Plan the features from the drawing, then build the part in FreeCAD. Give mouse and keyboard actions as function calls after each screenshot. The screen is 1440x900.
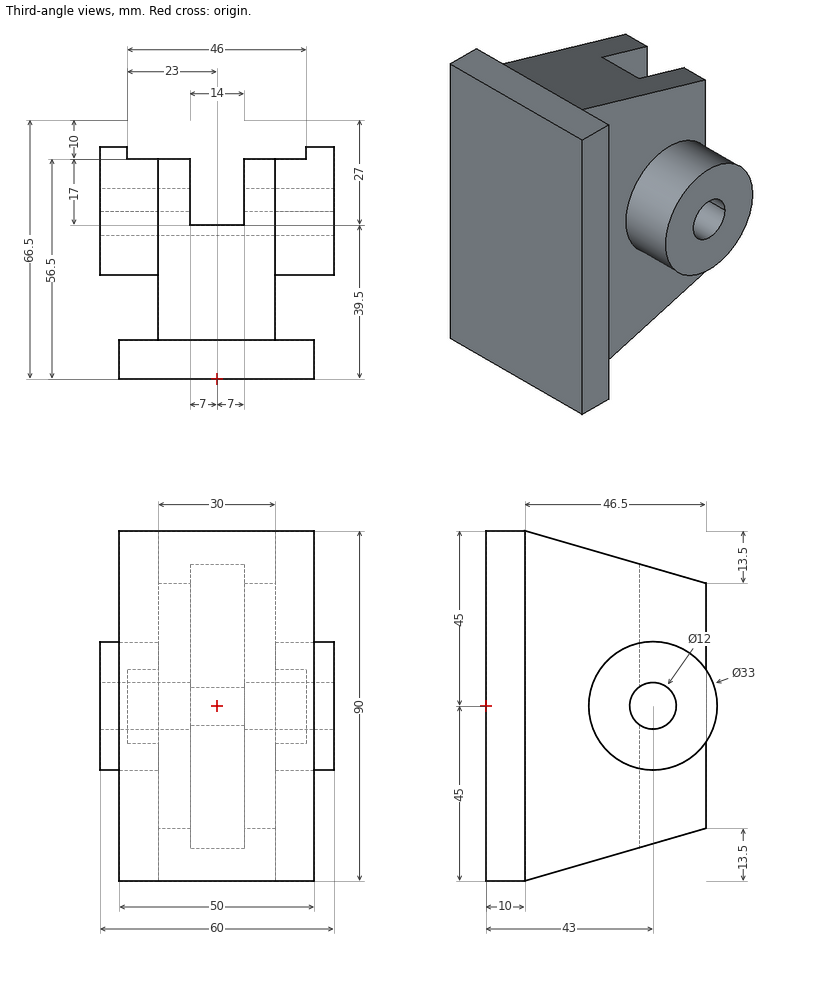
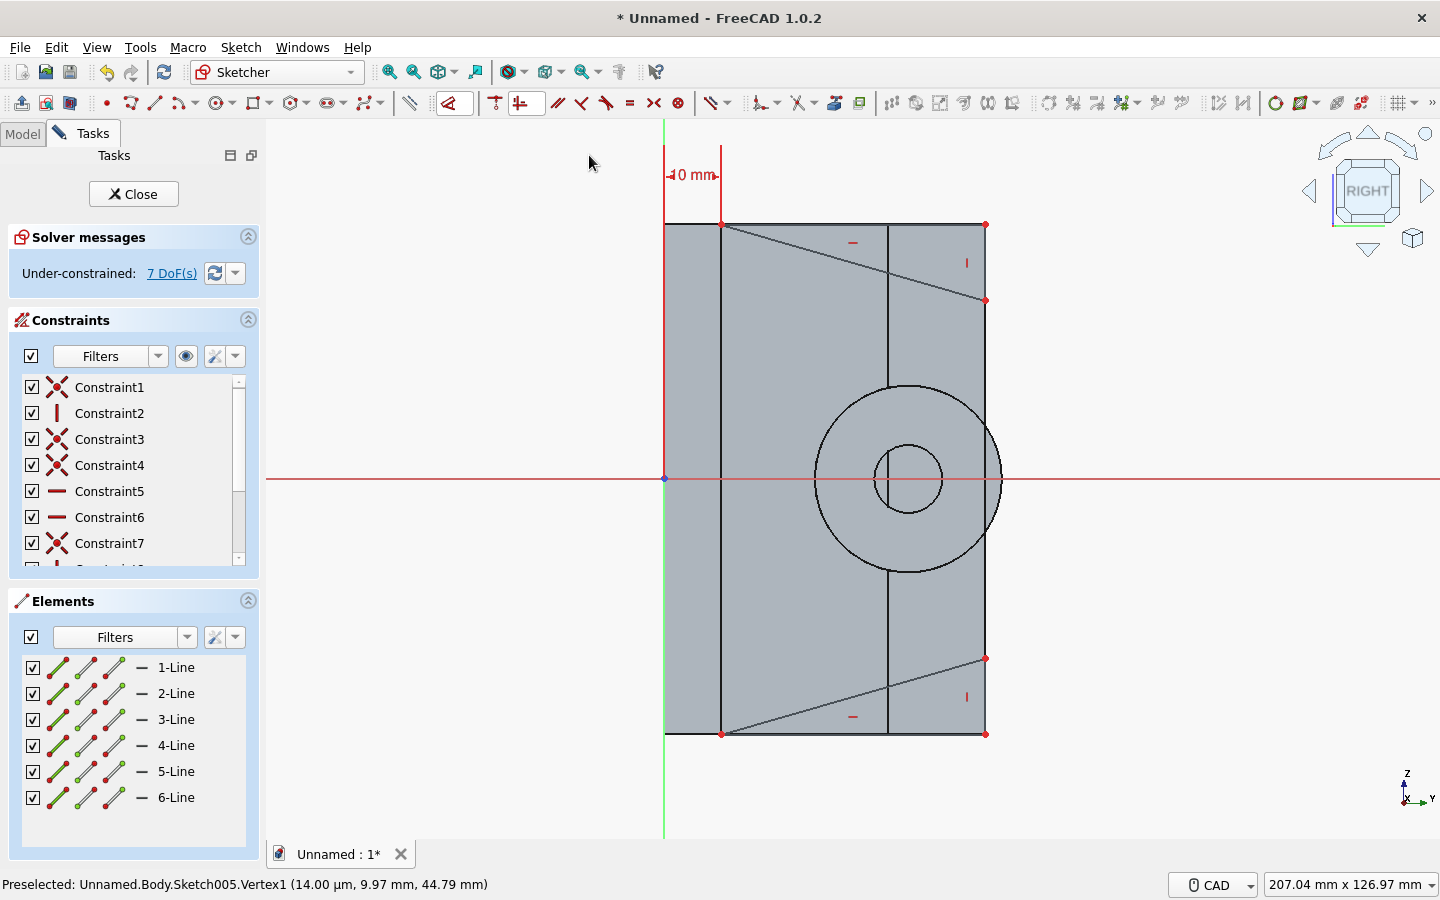
click(721, 225)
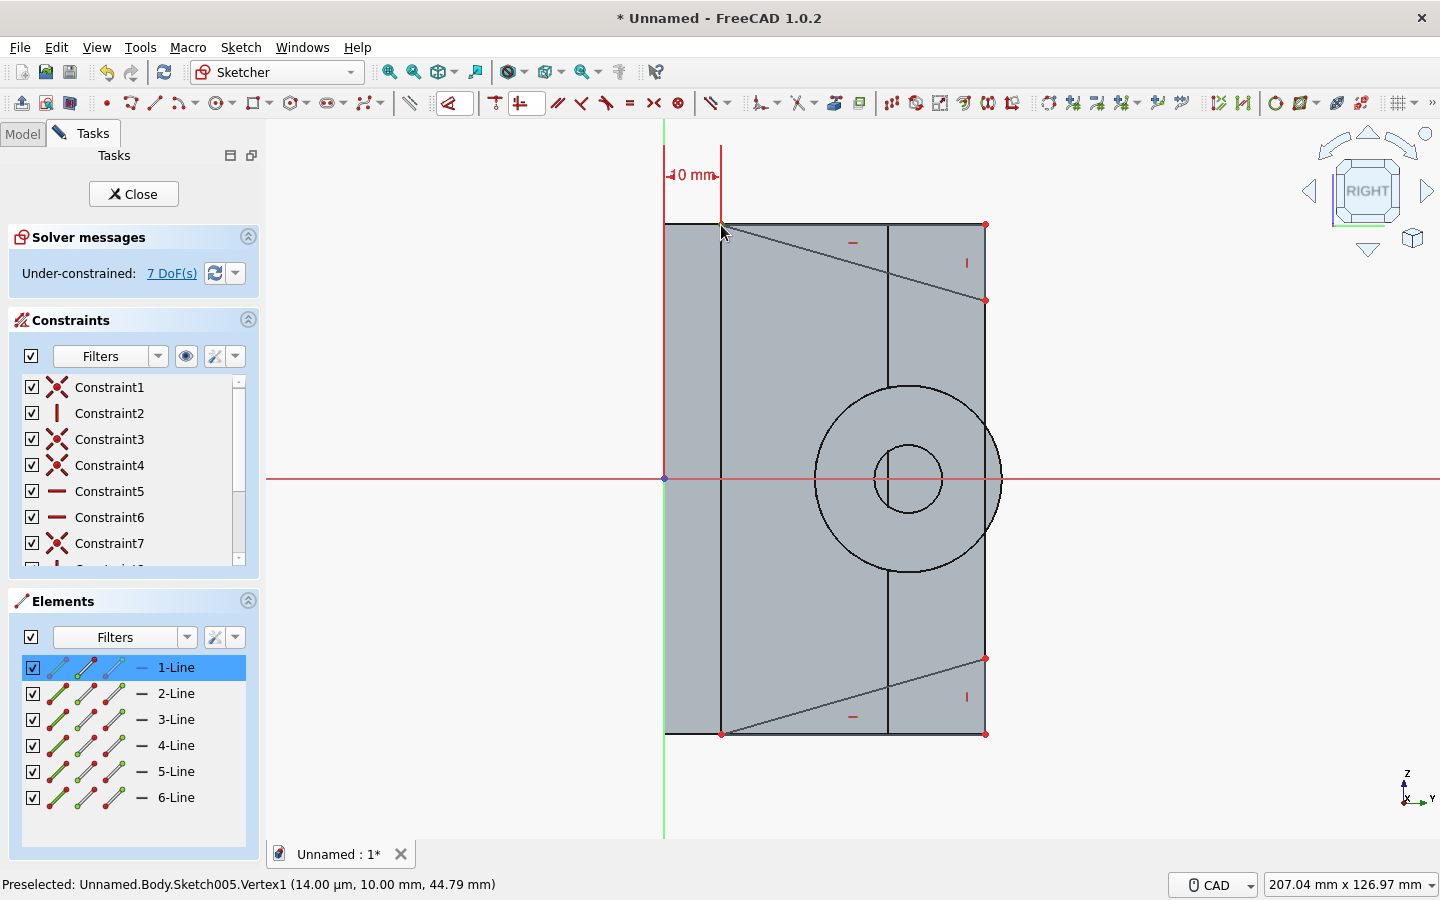
click(468, 104)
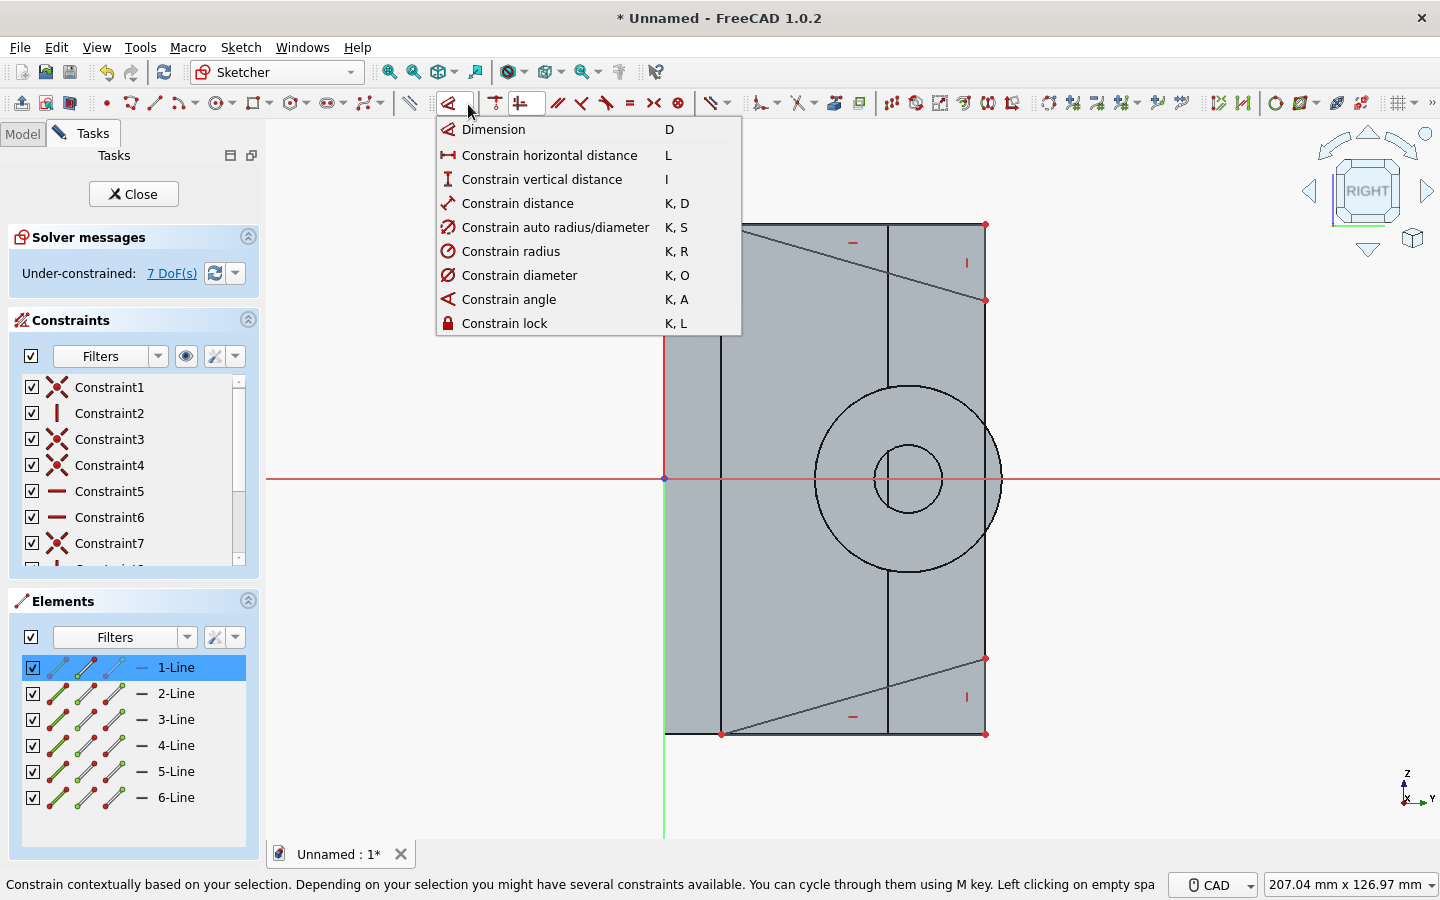
click(589, 179)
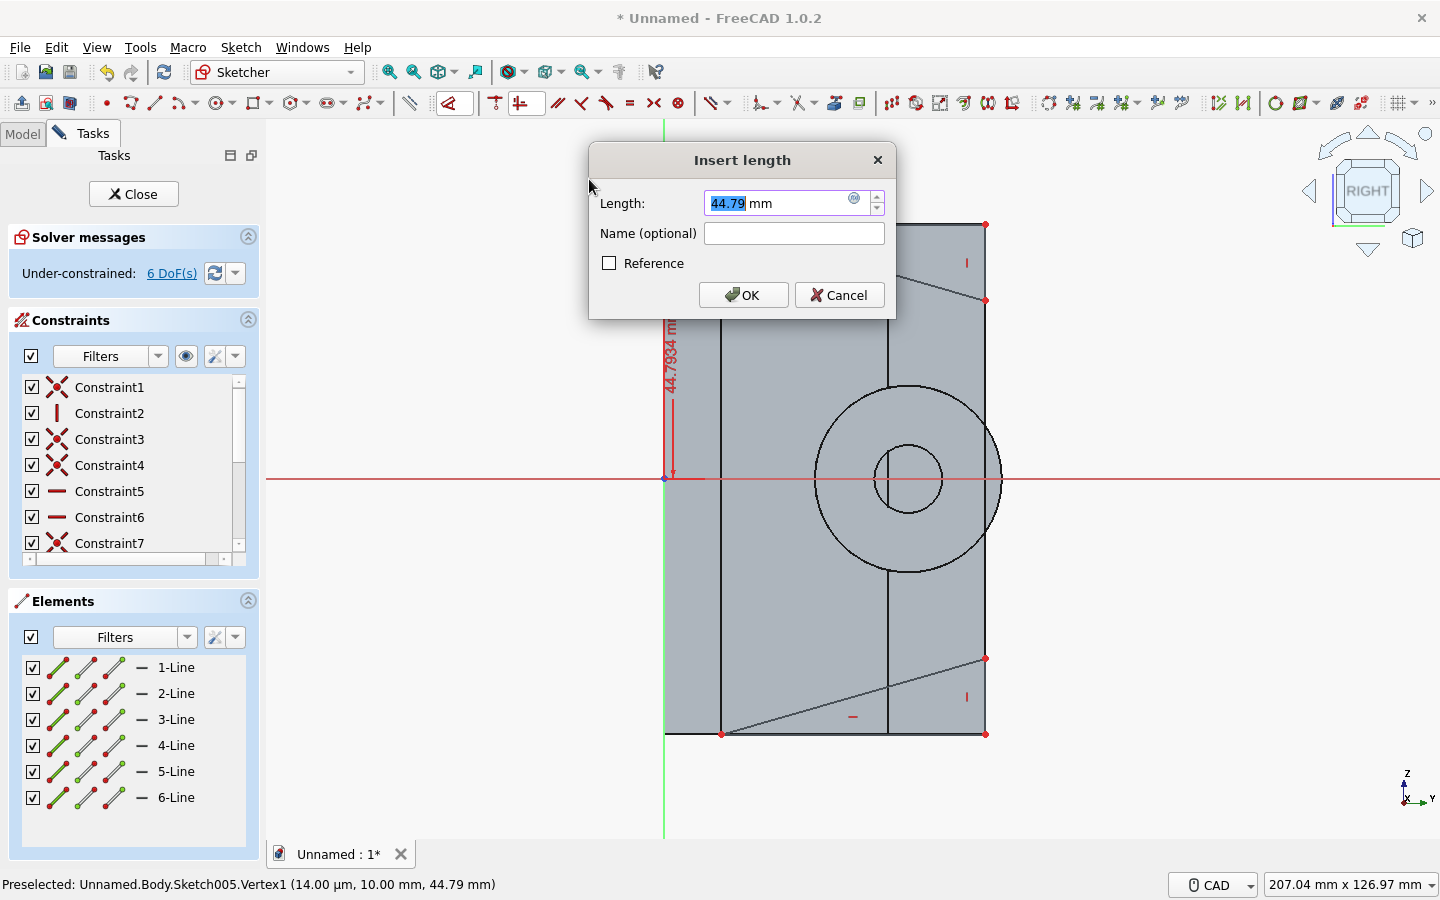
text(45)
key(Return)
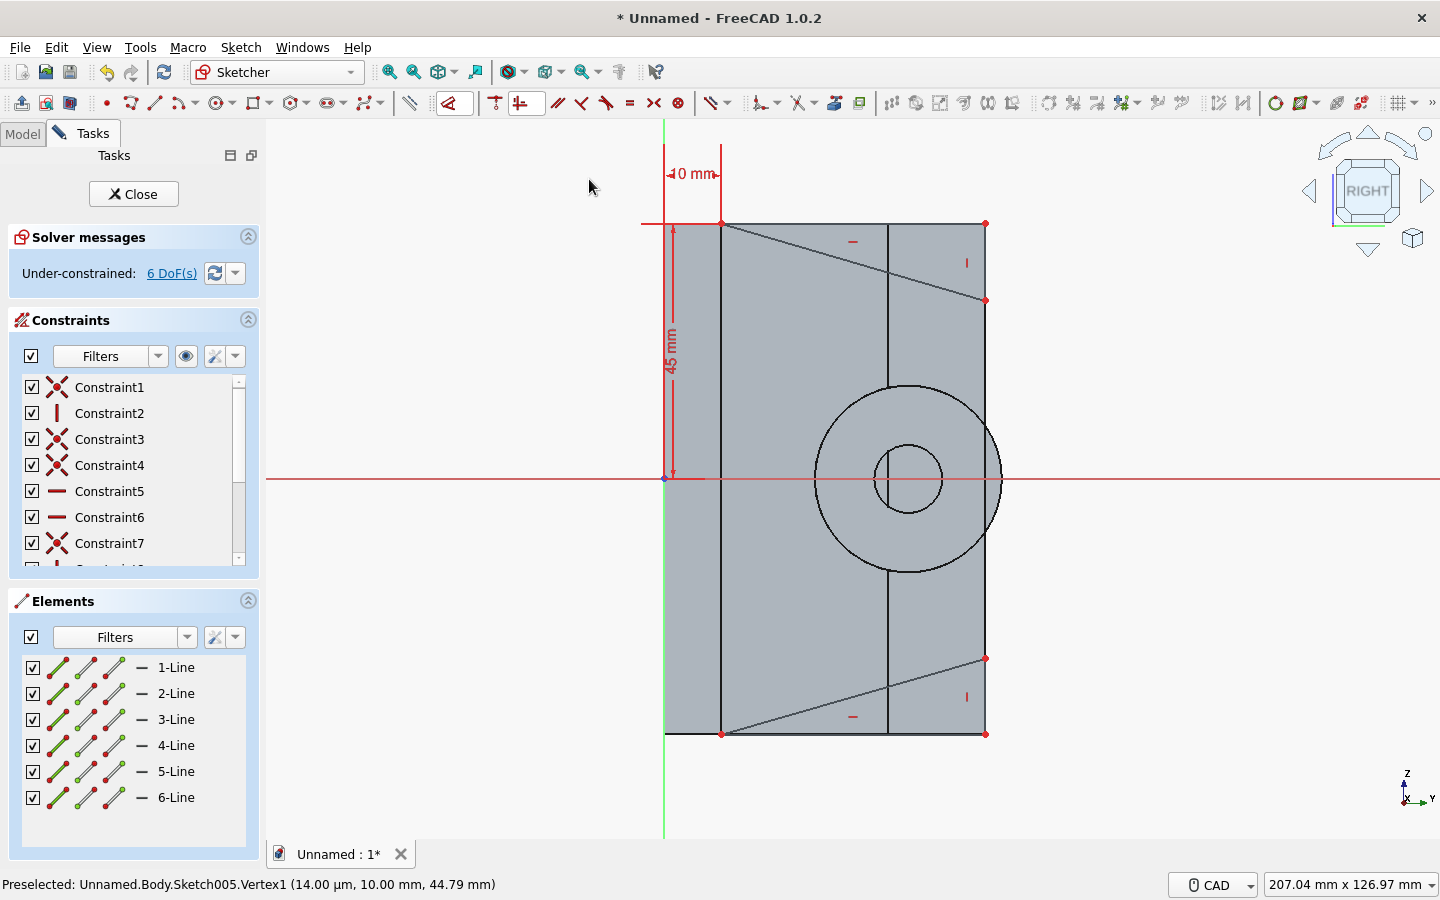
click(721, 735)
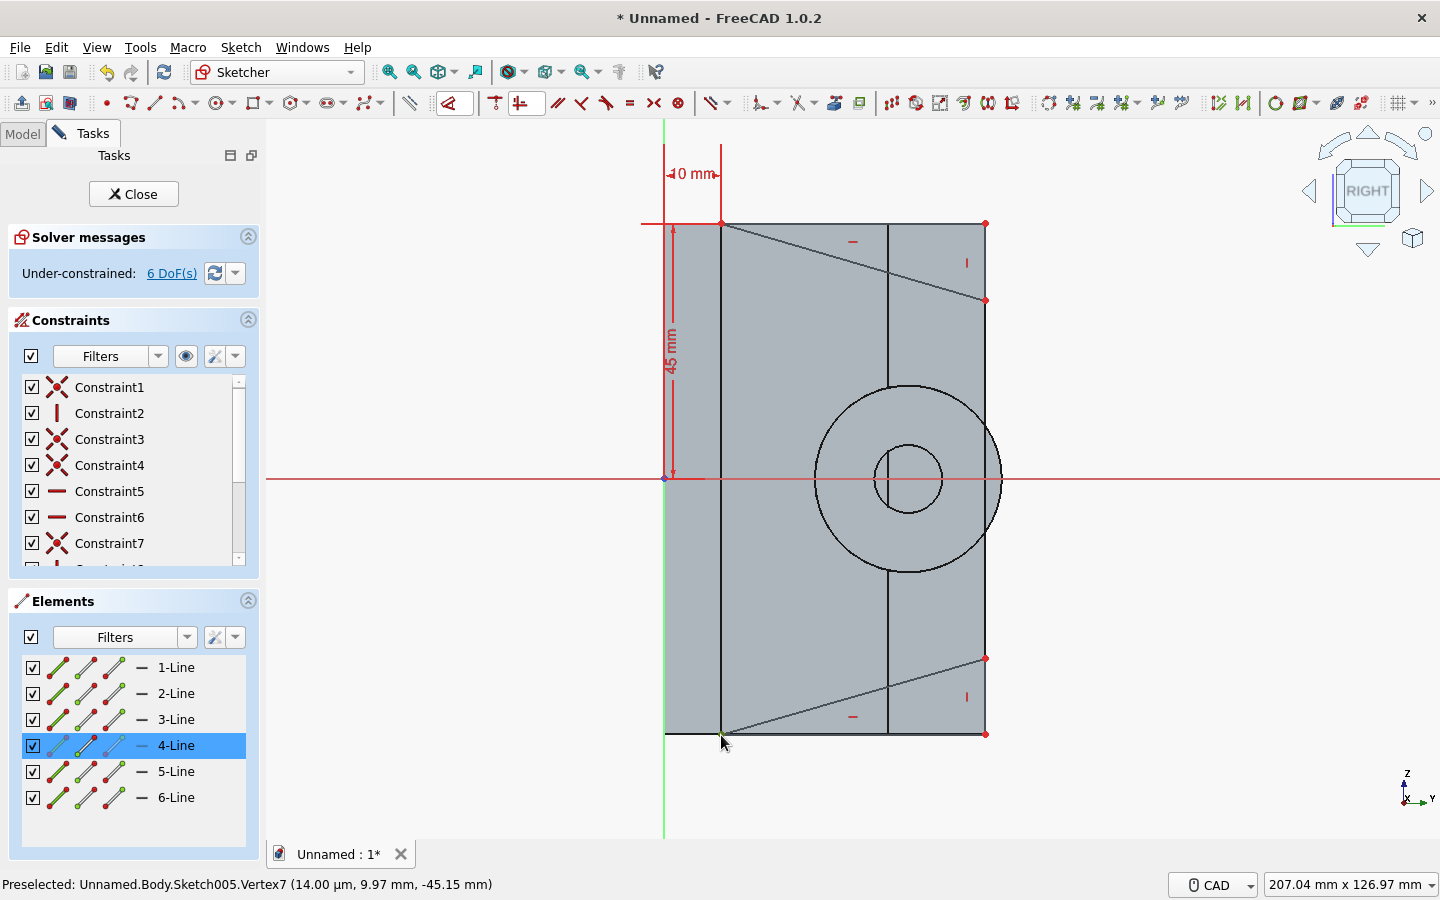
key(l)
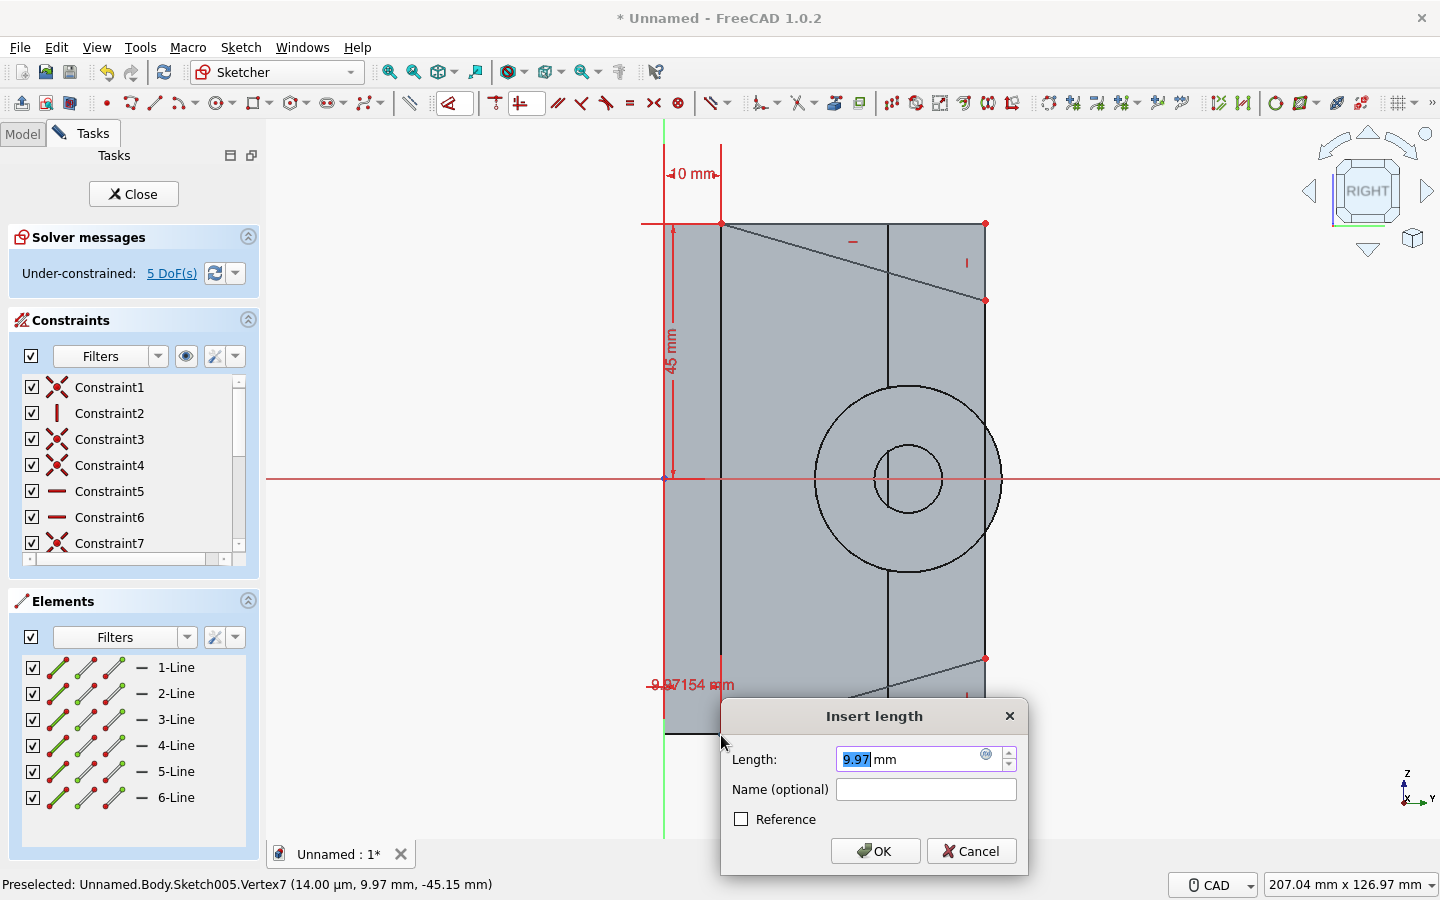
text(10)
key(Return)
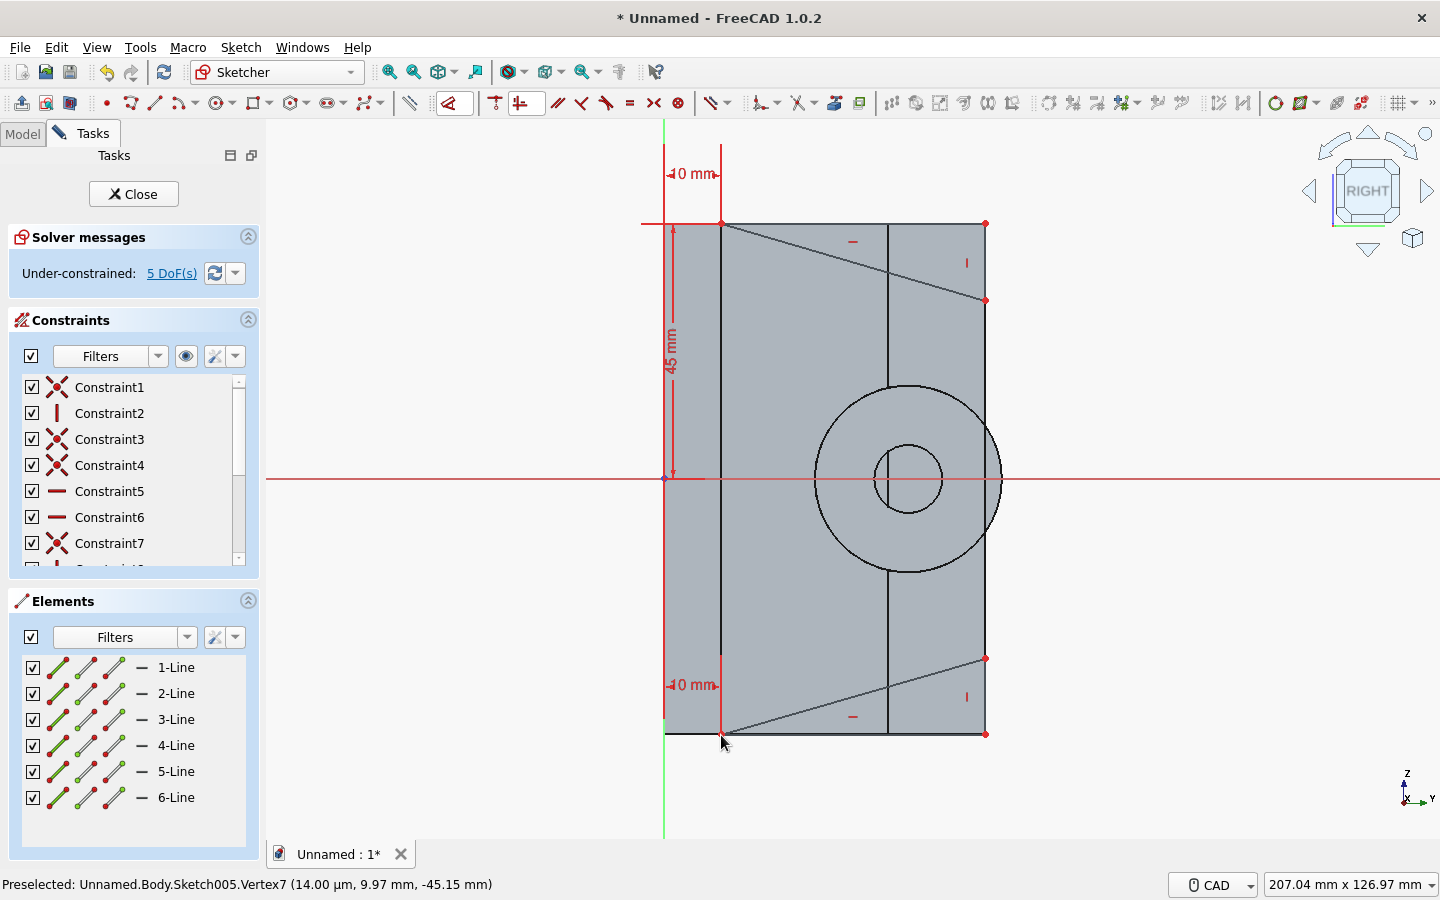
click(721, 735)